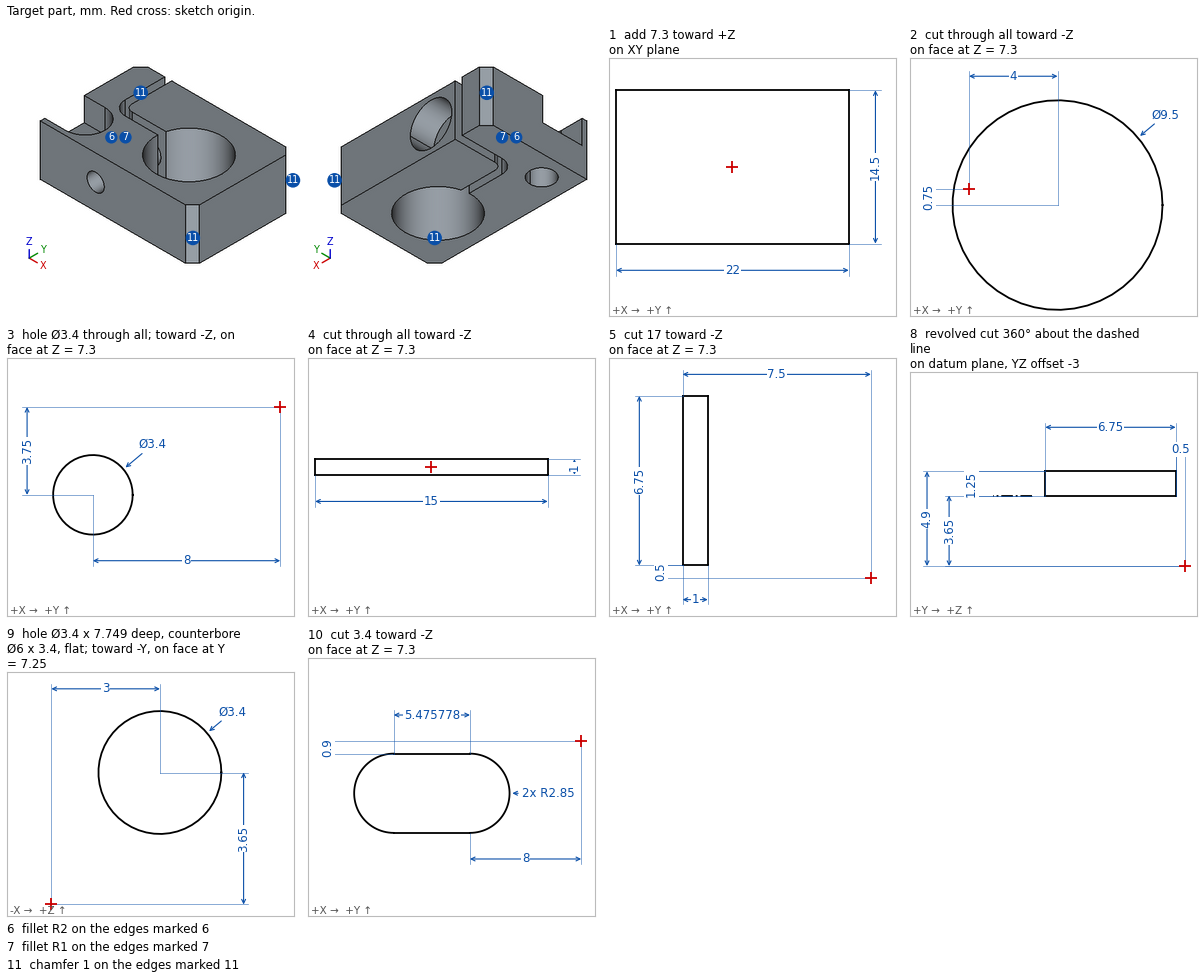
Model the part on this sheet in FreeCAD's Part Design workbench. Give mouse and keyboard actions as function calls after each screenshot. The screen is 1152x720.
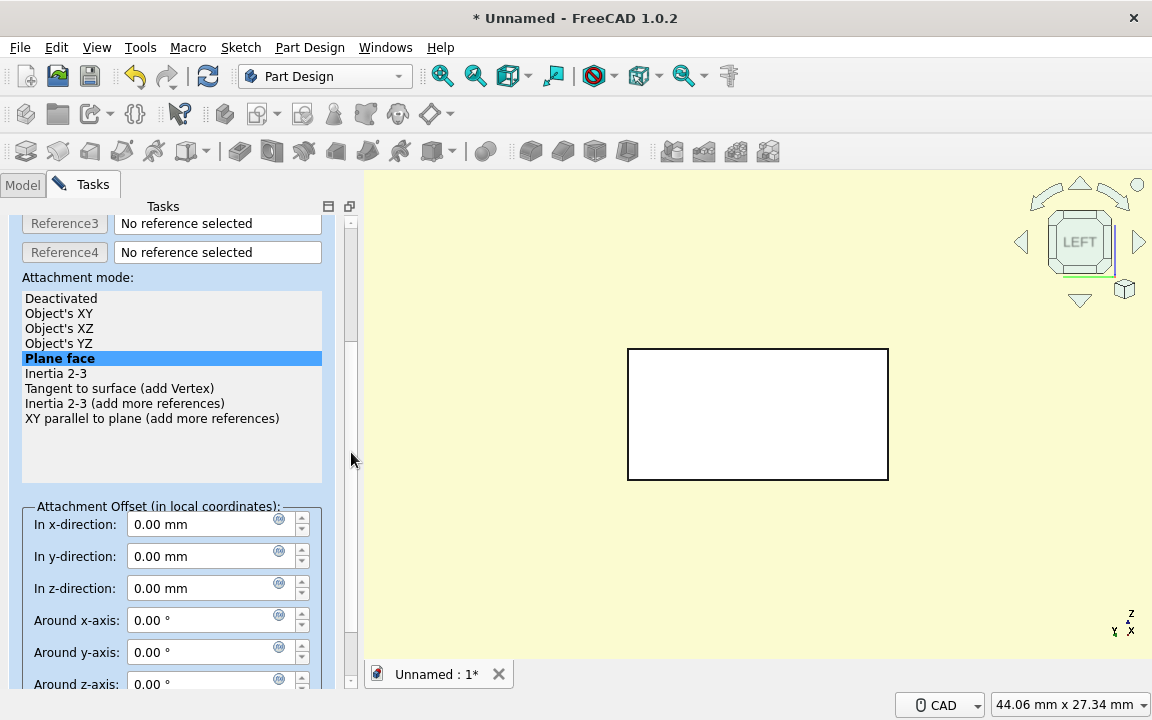
triple_click(210, 588)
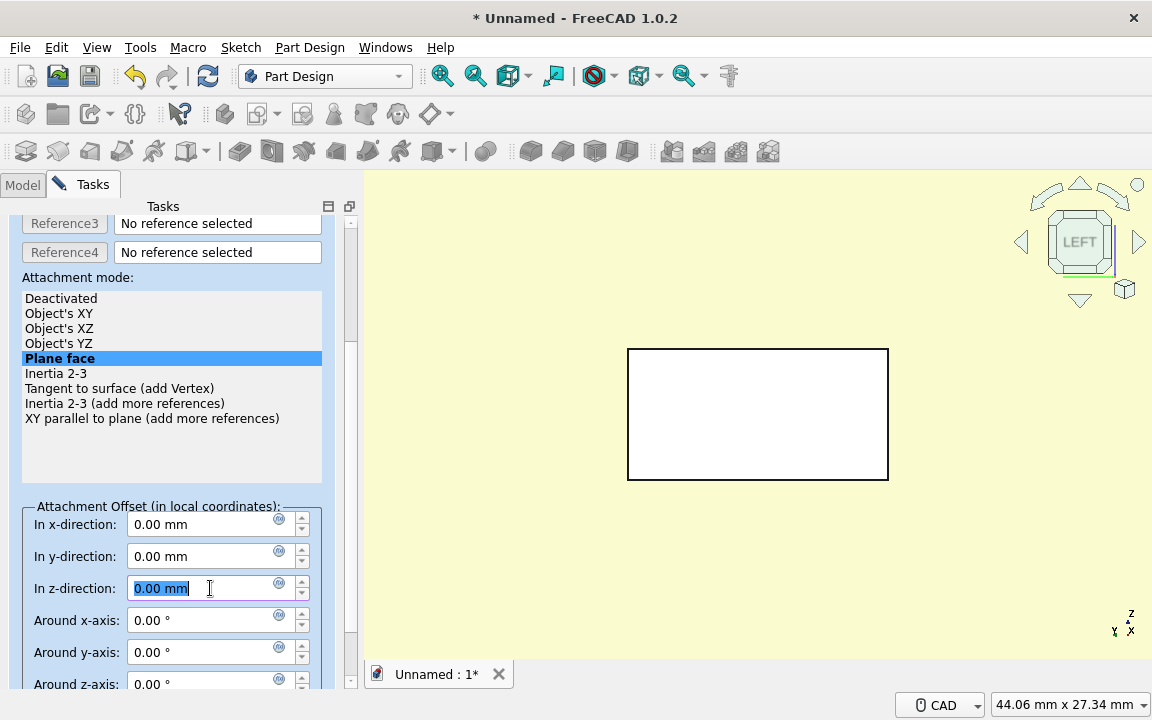
text(-3)
key(Tab)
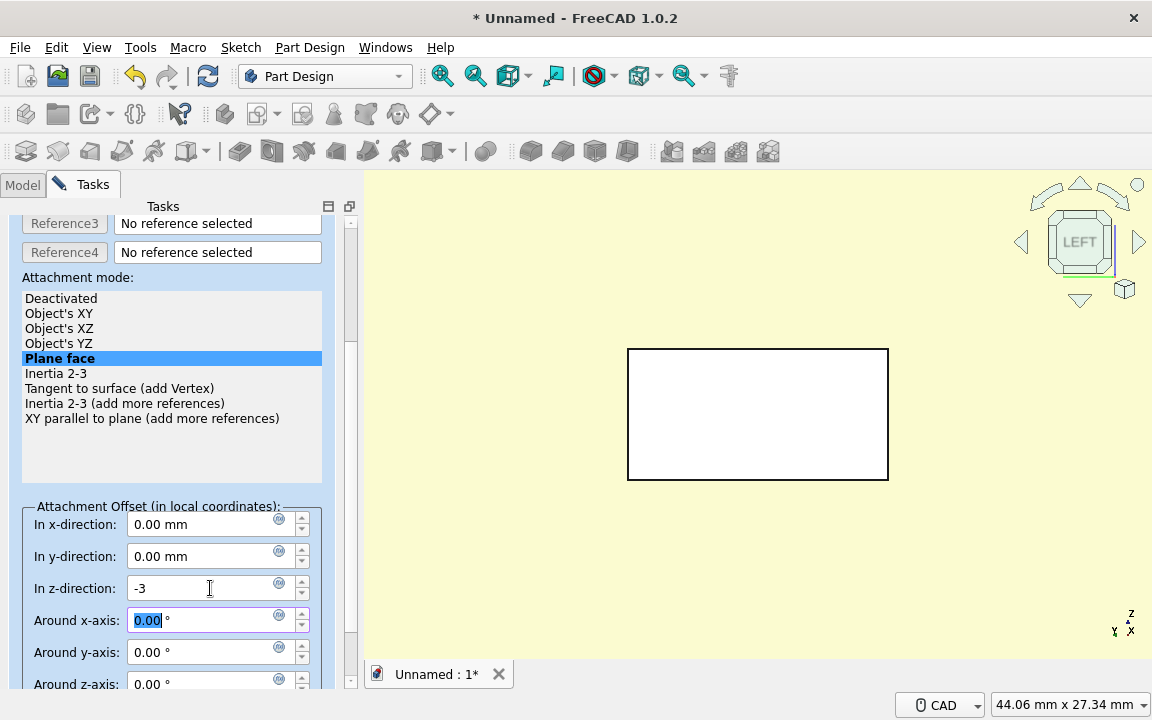
scroll(351, 452, up, 4)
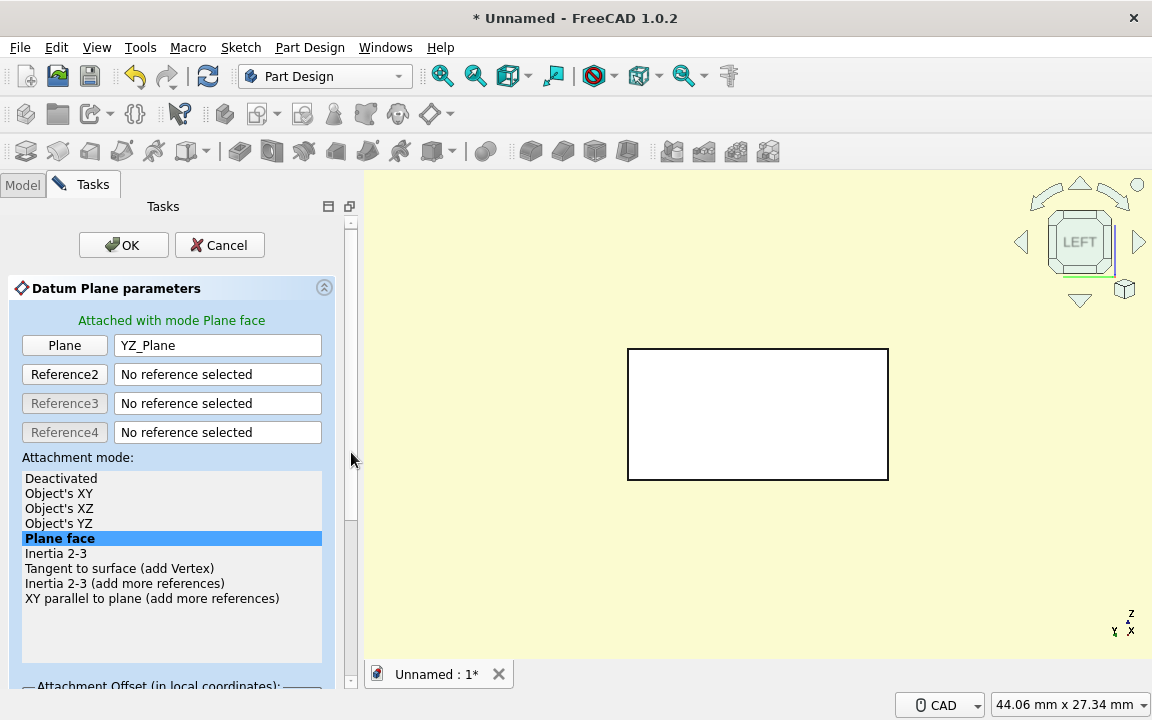
click(124, 245)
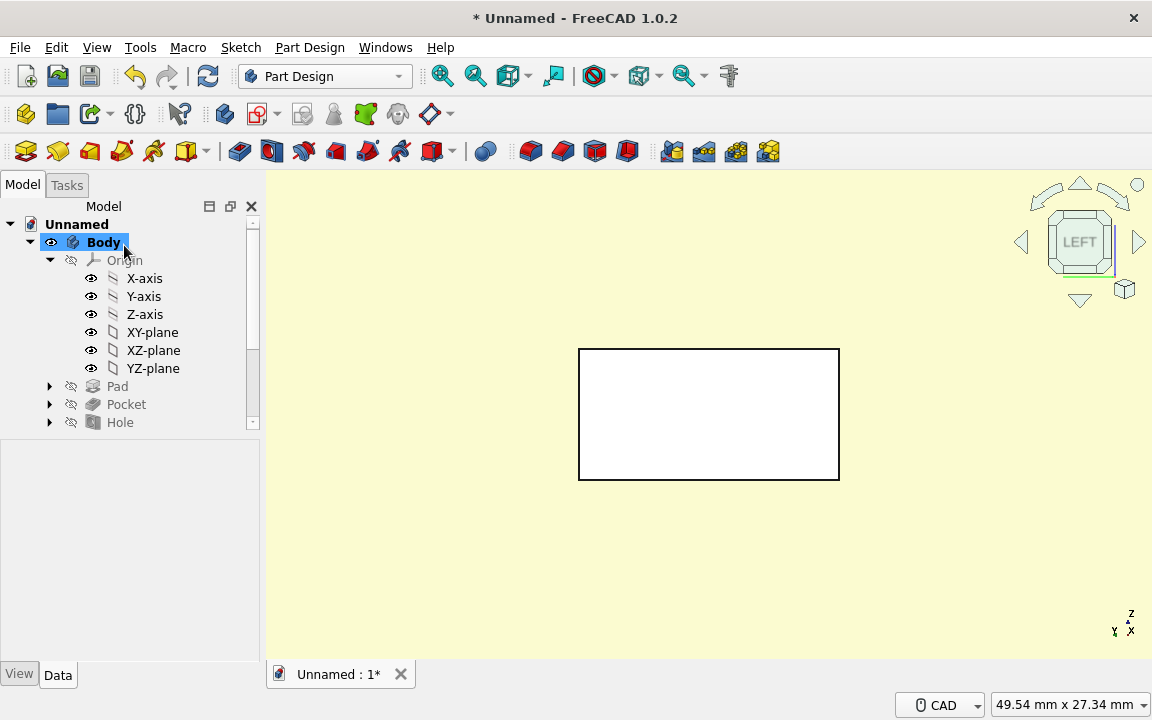
scroll(100, 328, down, 3)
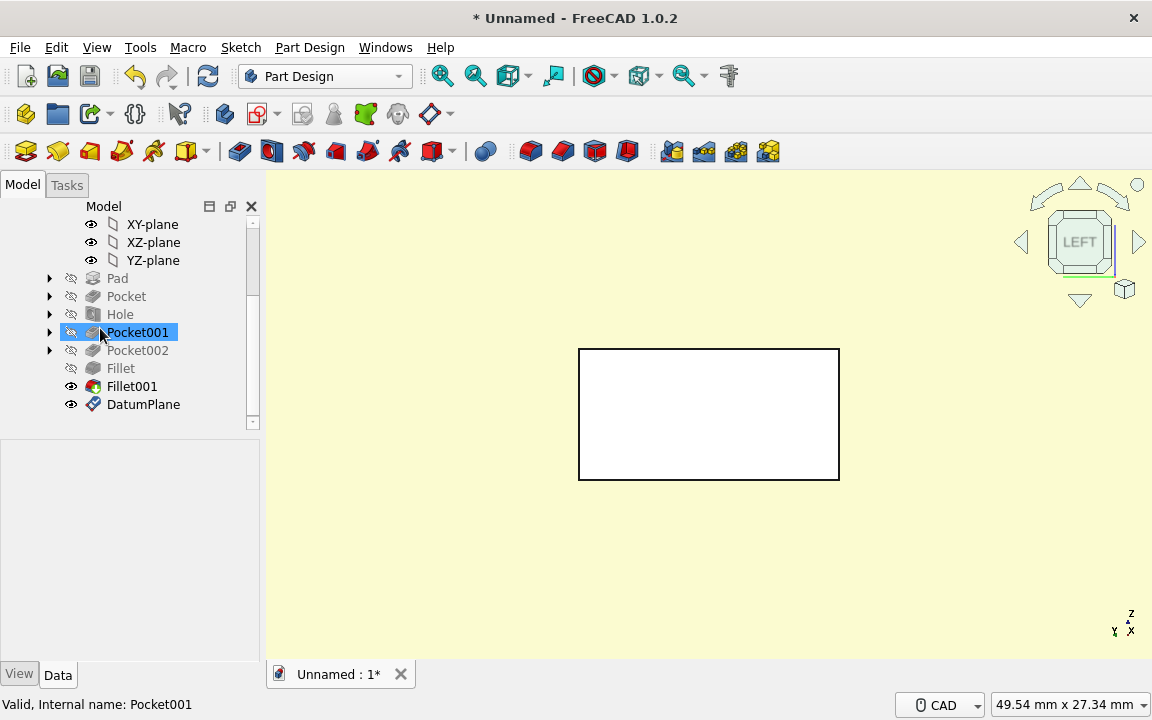
click(116, 404)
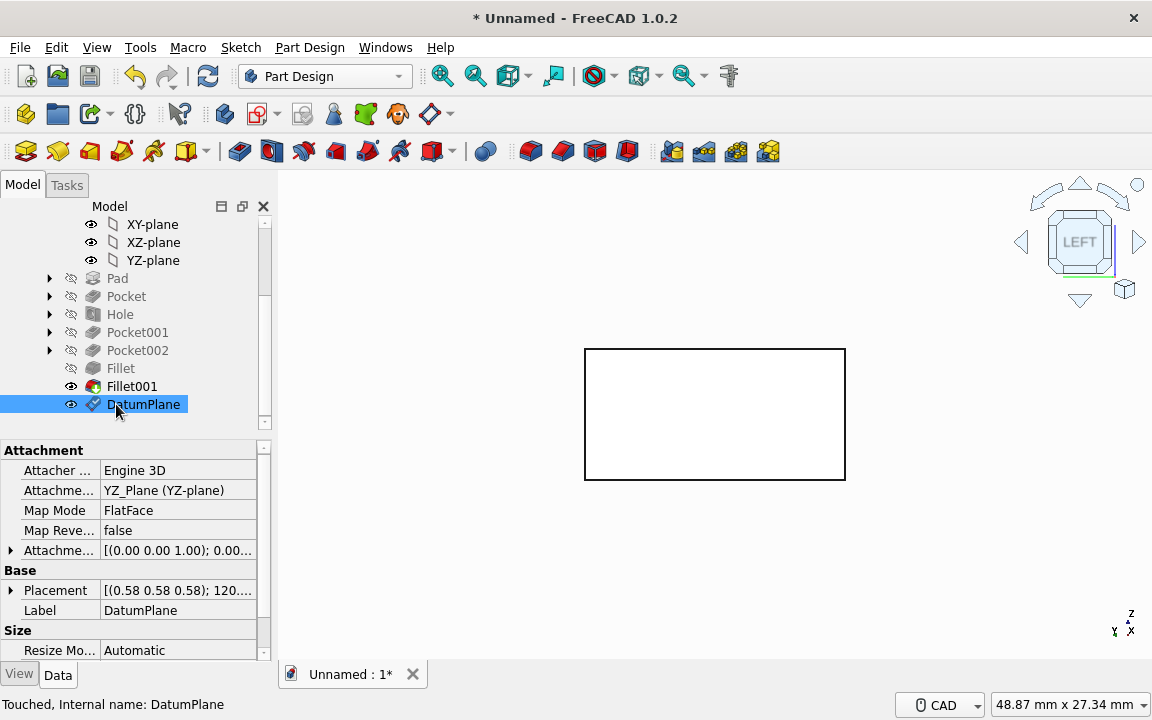
click(258, 114)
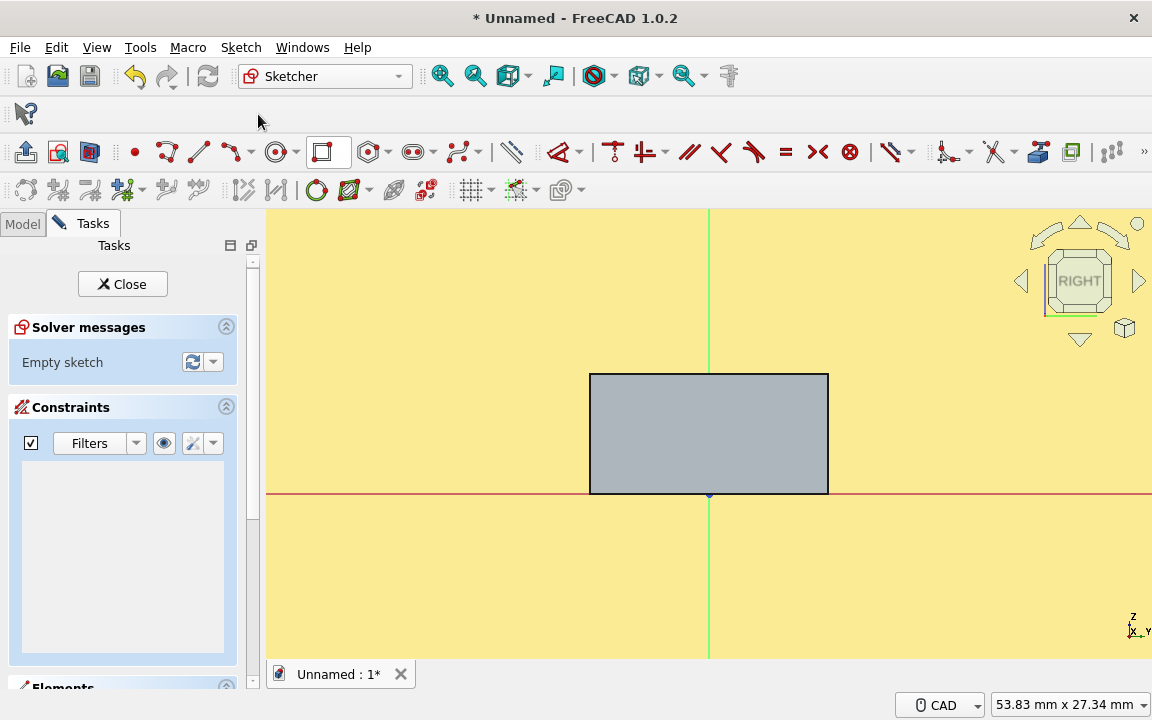
click(90, 152)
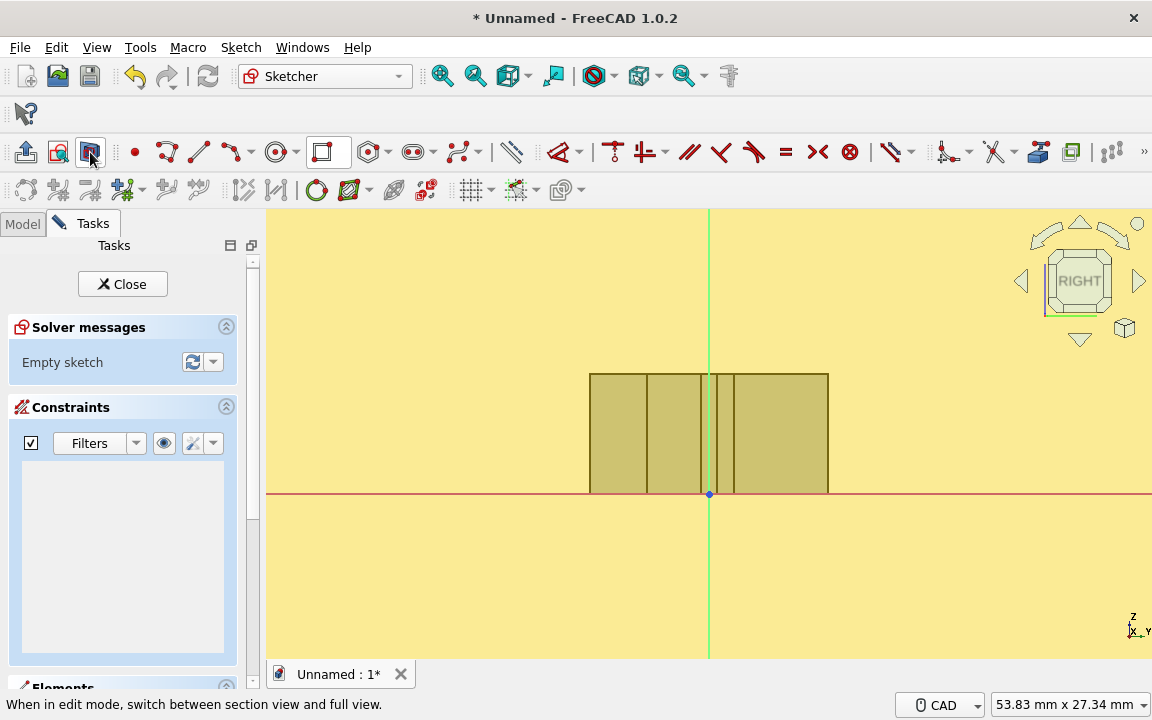
scroll(619, 465, up, 5)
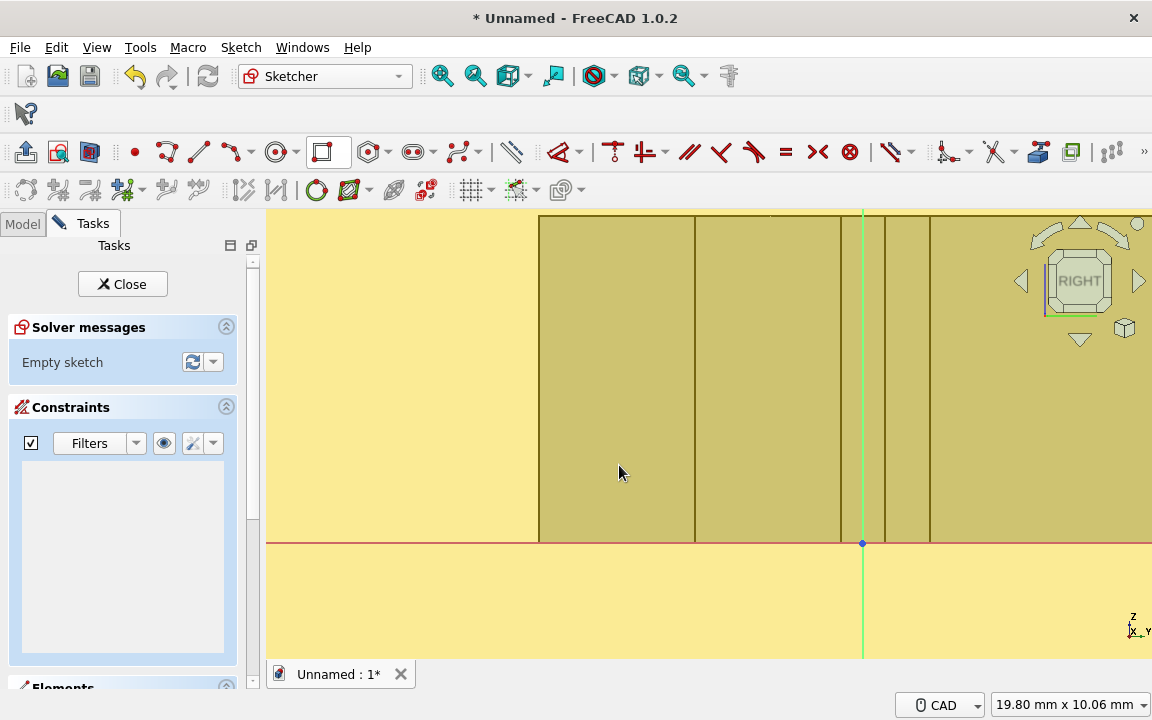
click(322, 152)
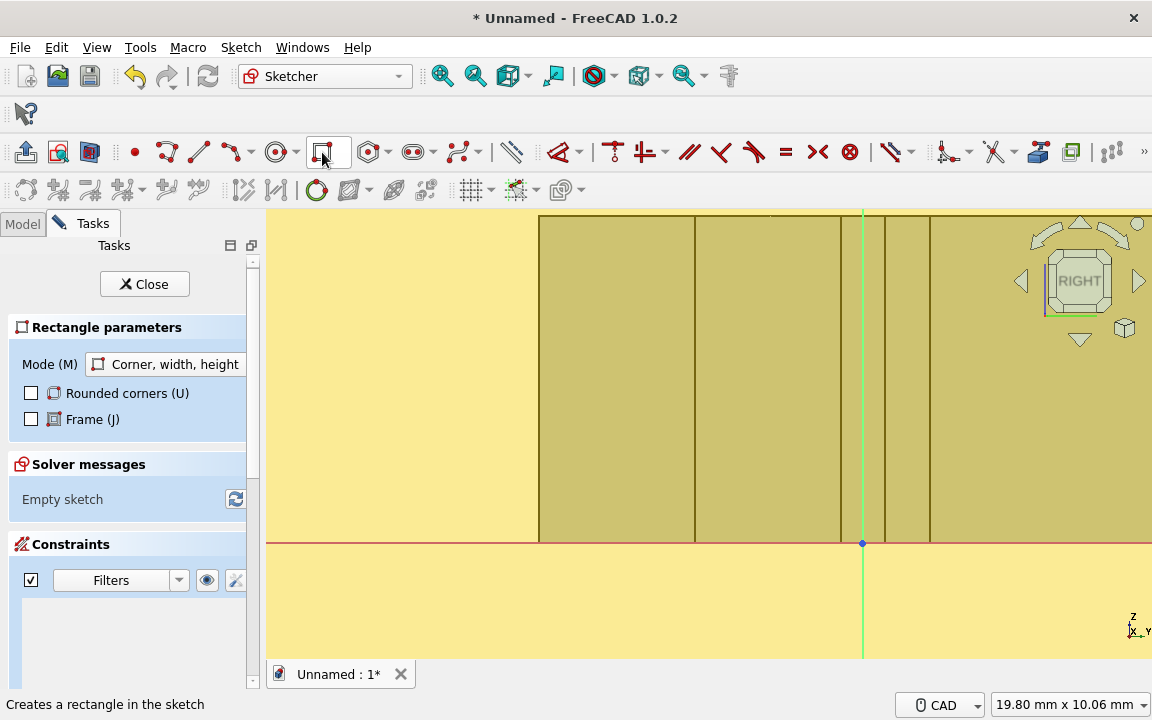
click(539, 324)
click(841, 380)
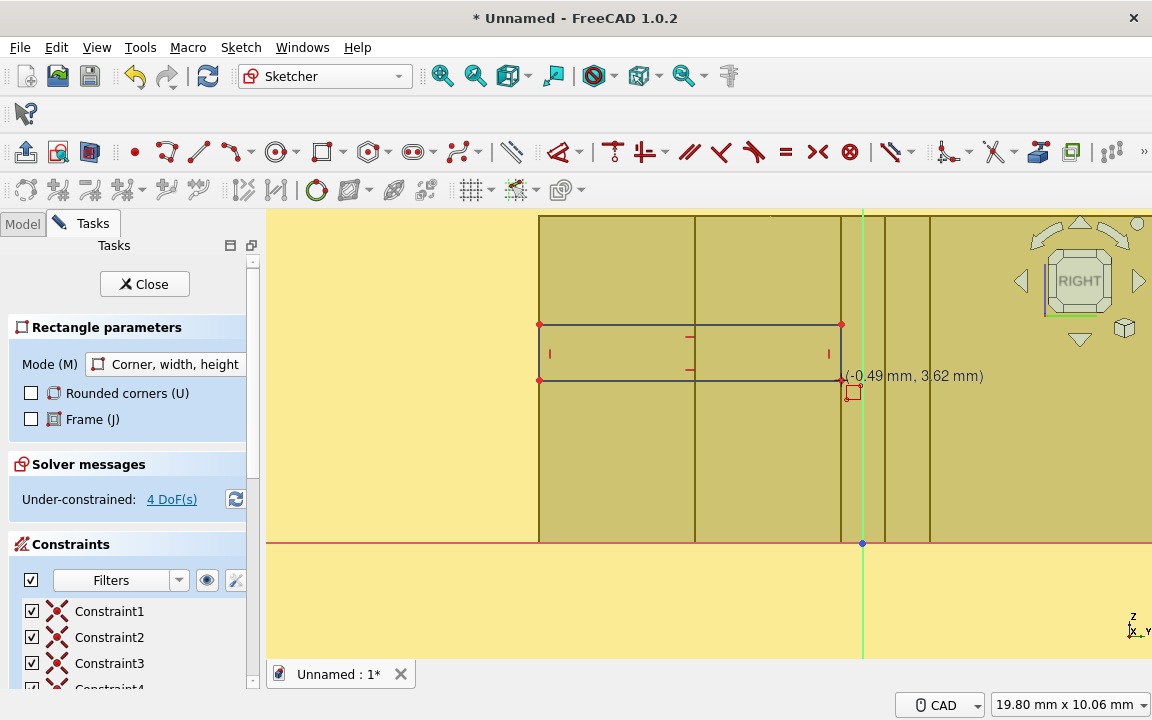
click(200, 152)